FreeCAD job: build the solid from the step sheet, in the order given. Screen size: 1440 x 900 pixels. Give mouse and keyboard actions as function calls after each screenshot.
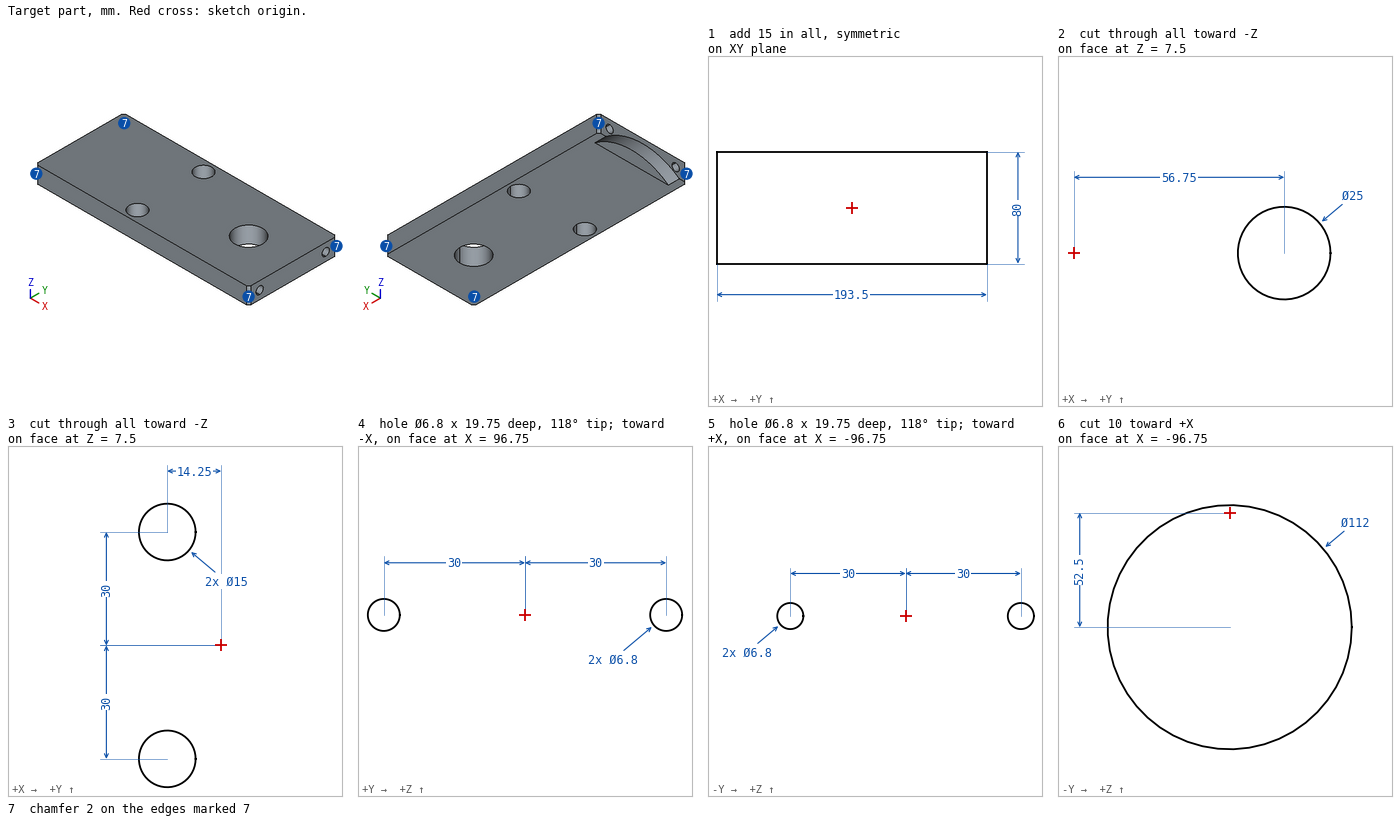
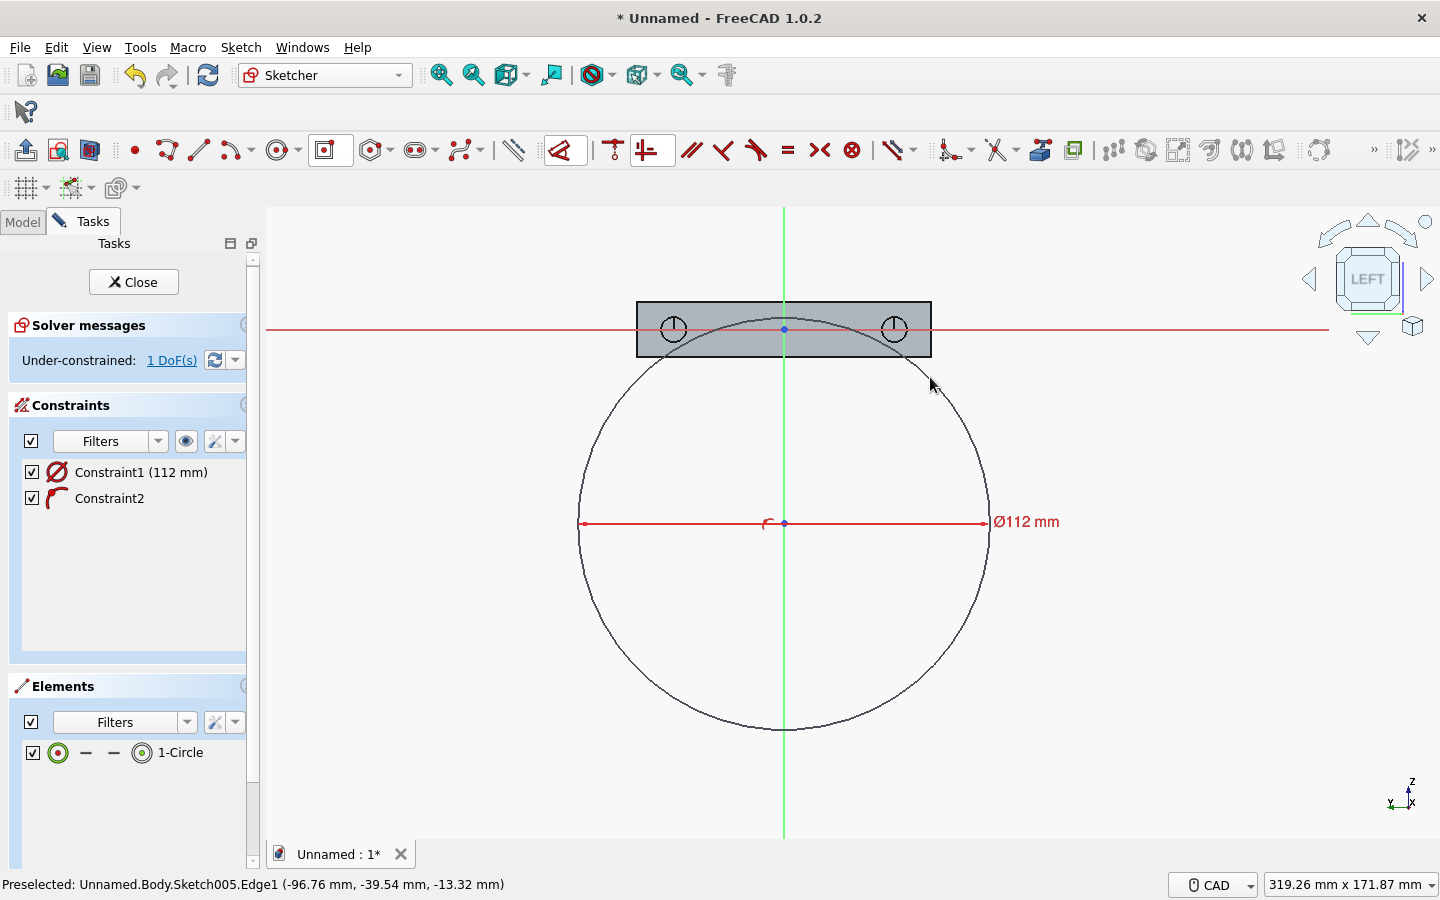
click(784, 524)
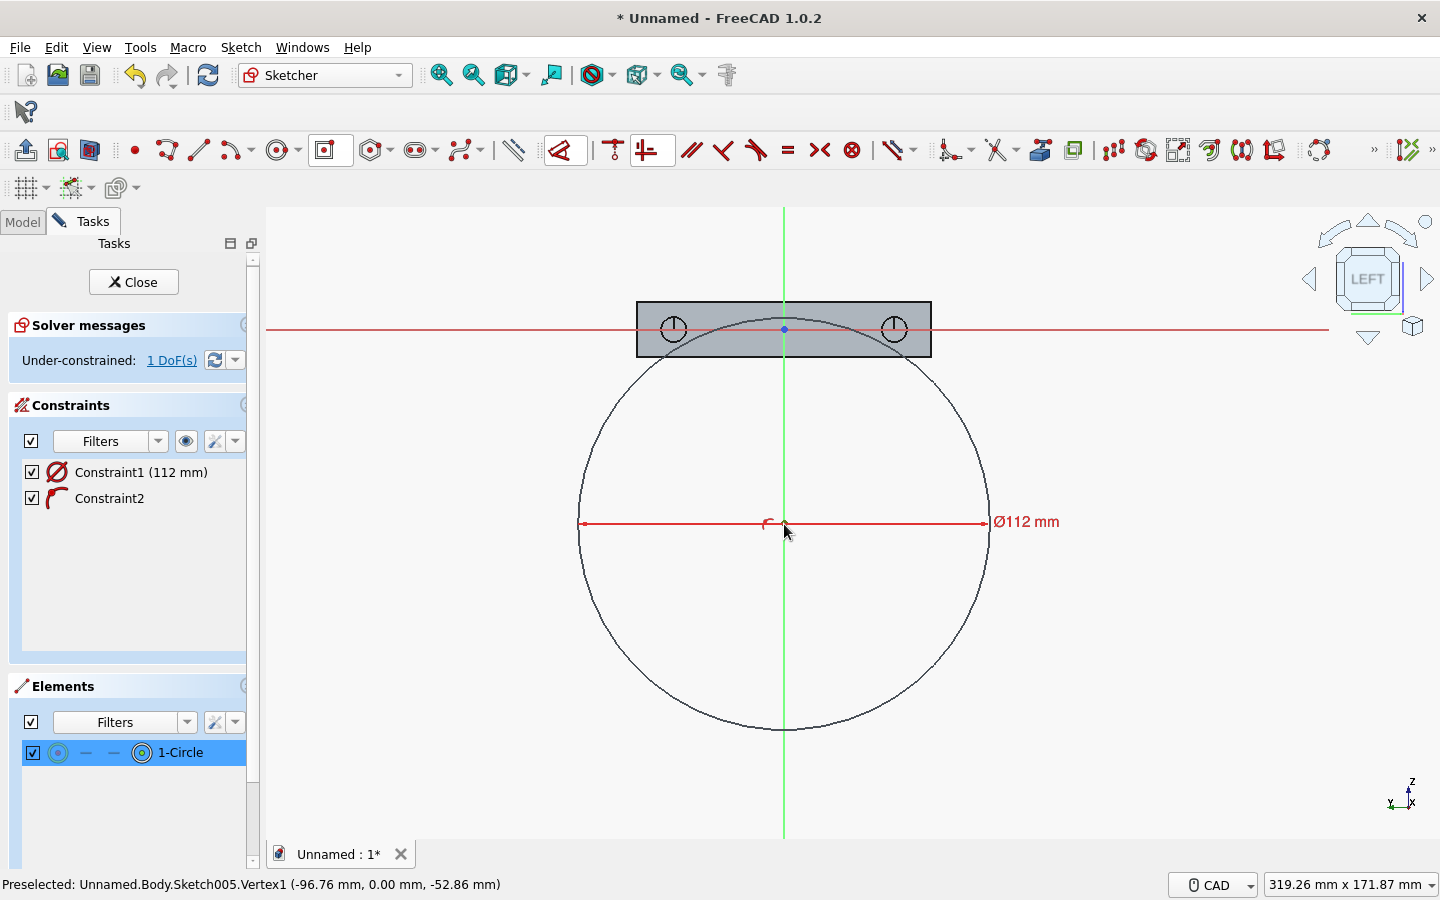
click(582, 150)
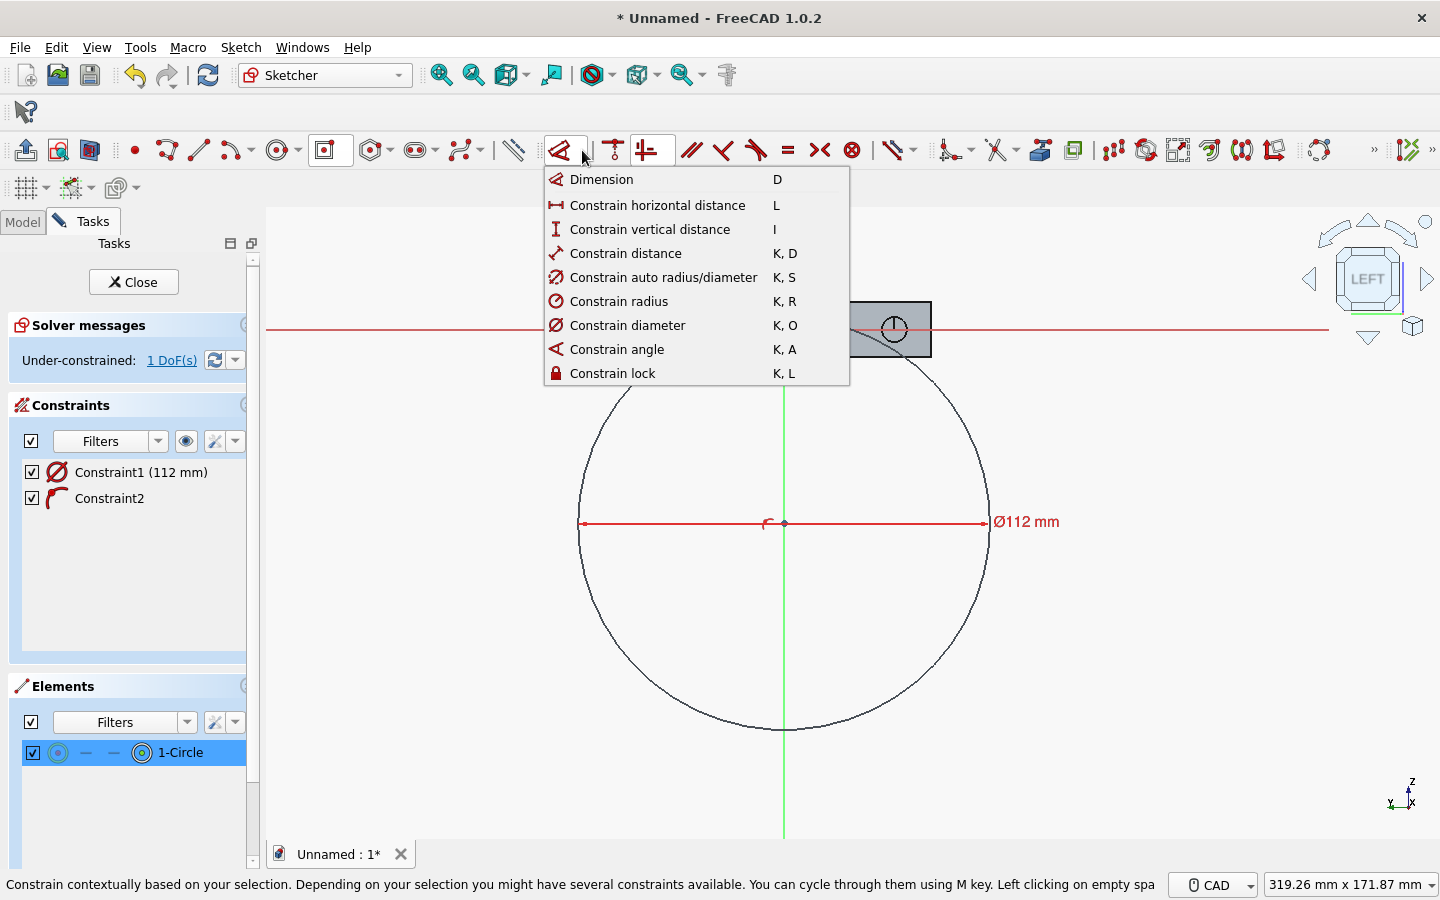
click(697, 229)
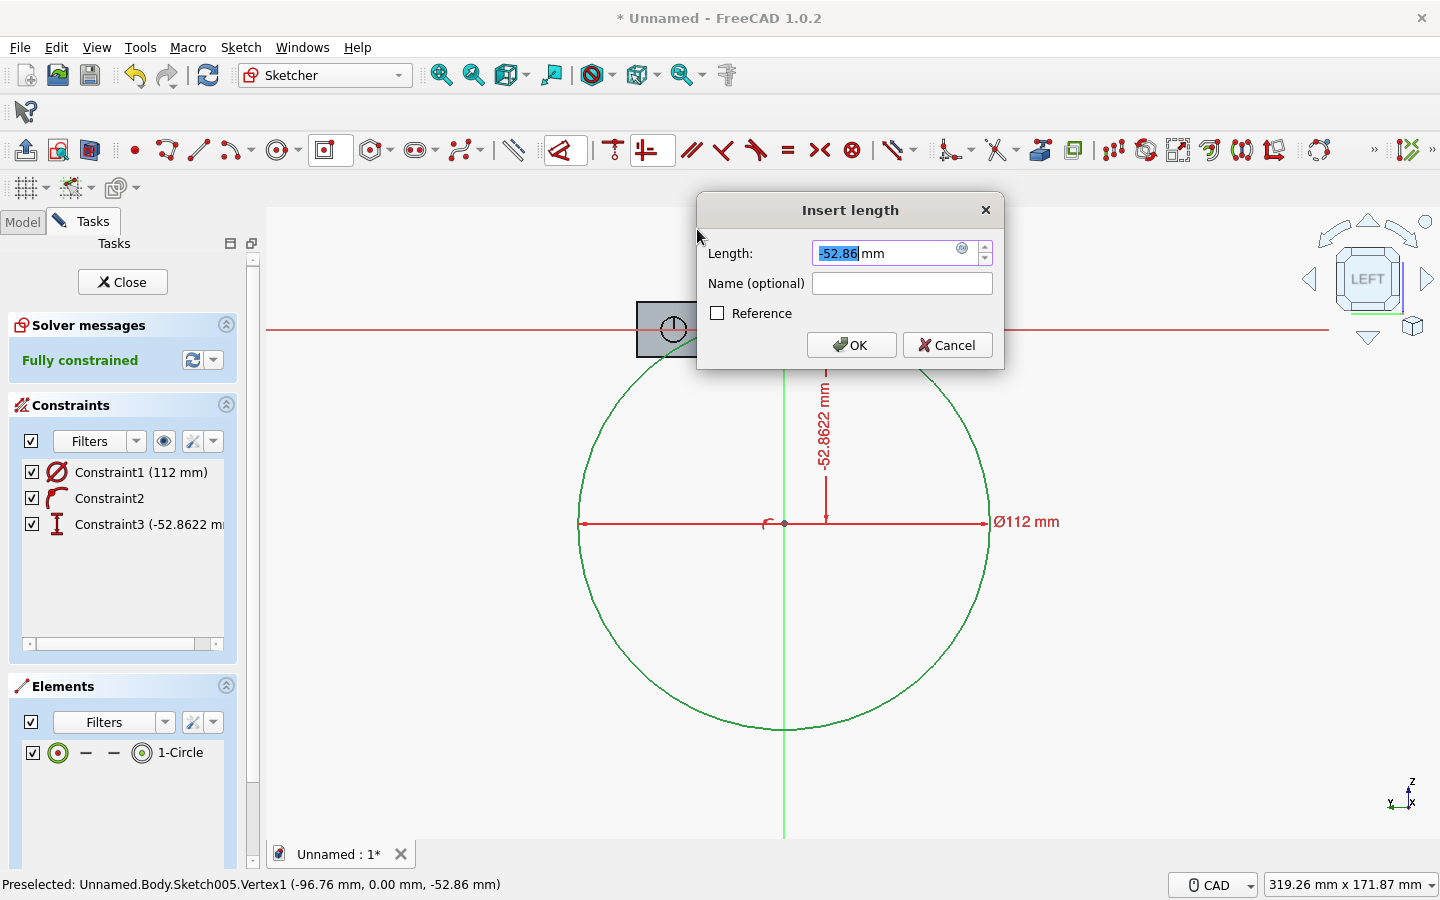
text(-52.5)
key(Return)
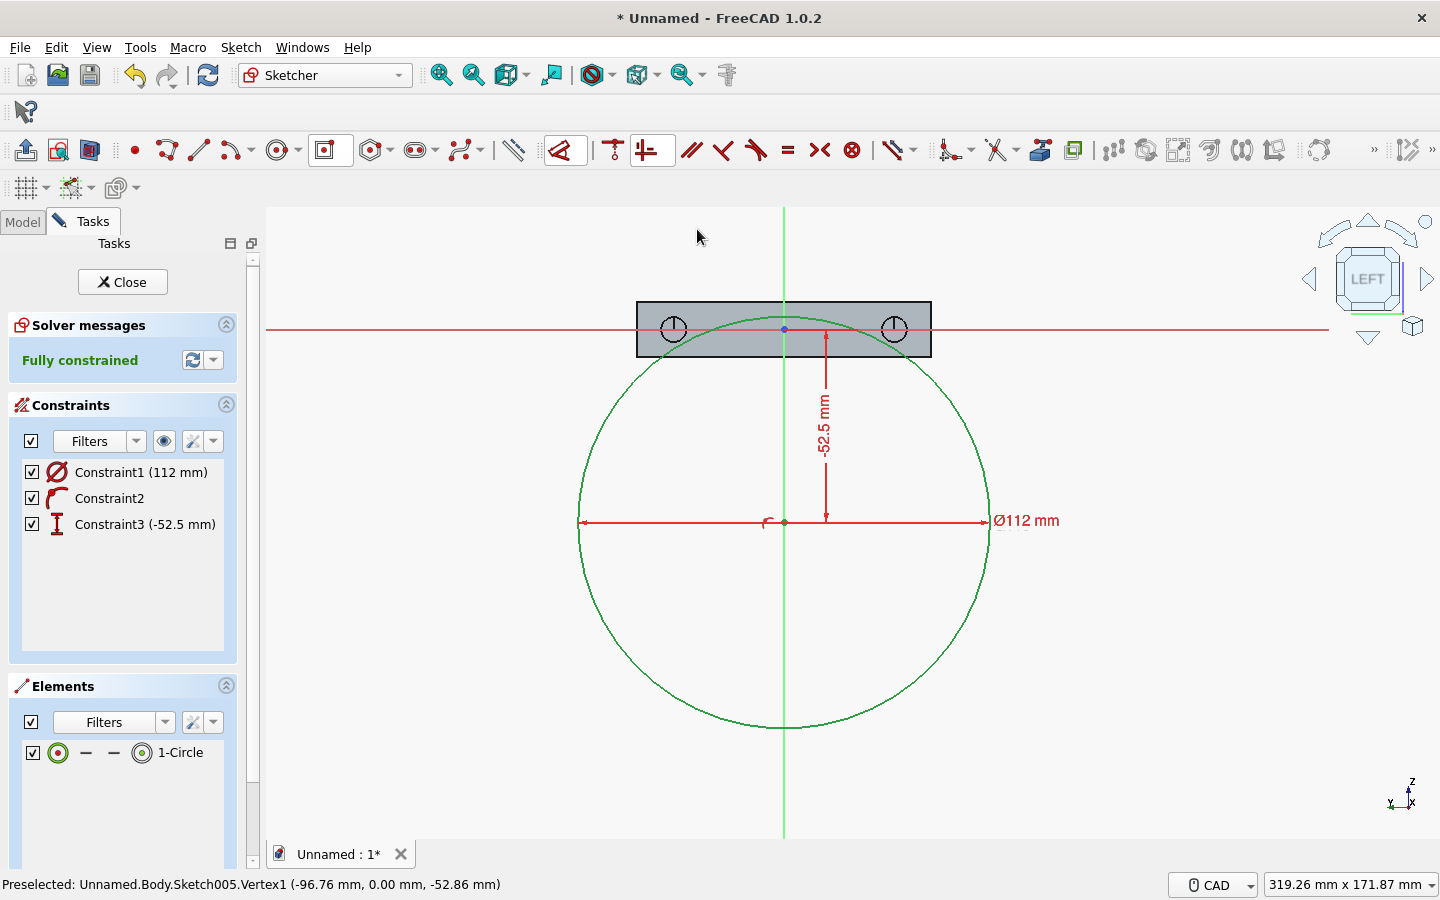
click(123, 282)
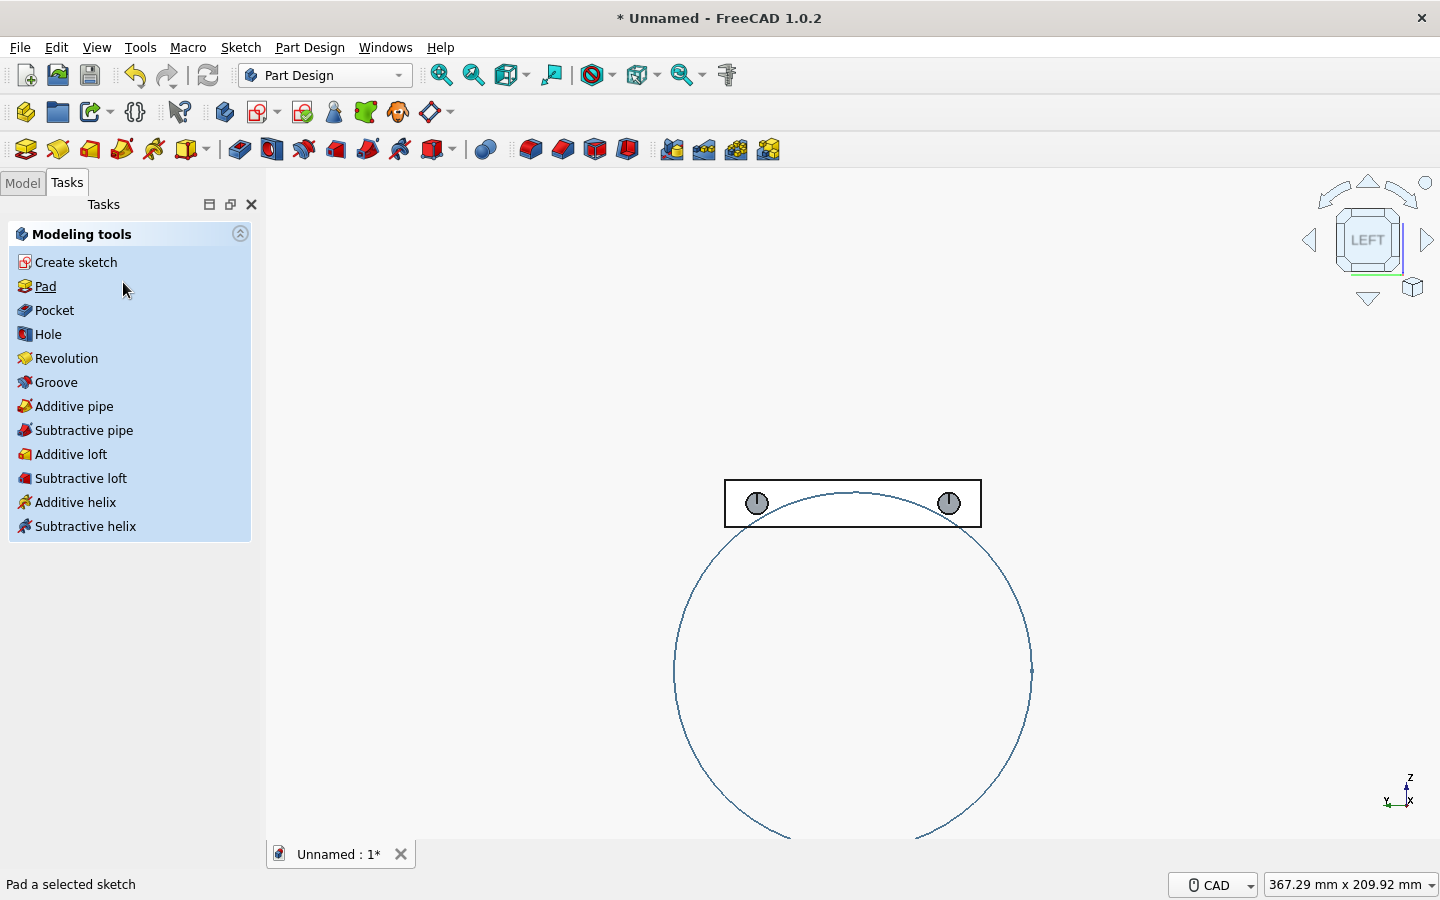
click(240, 150)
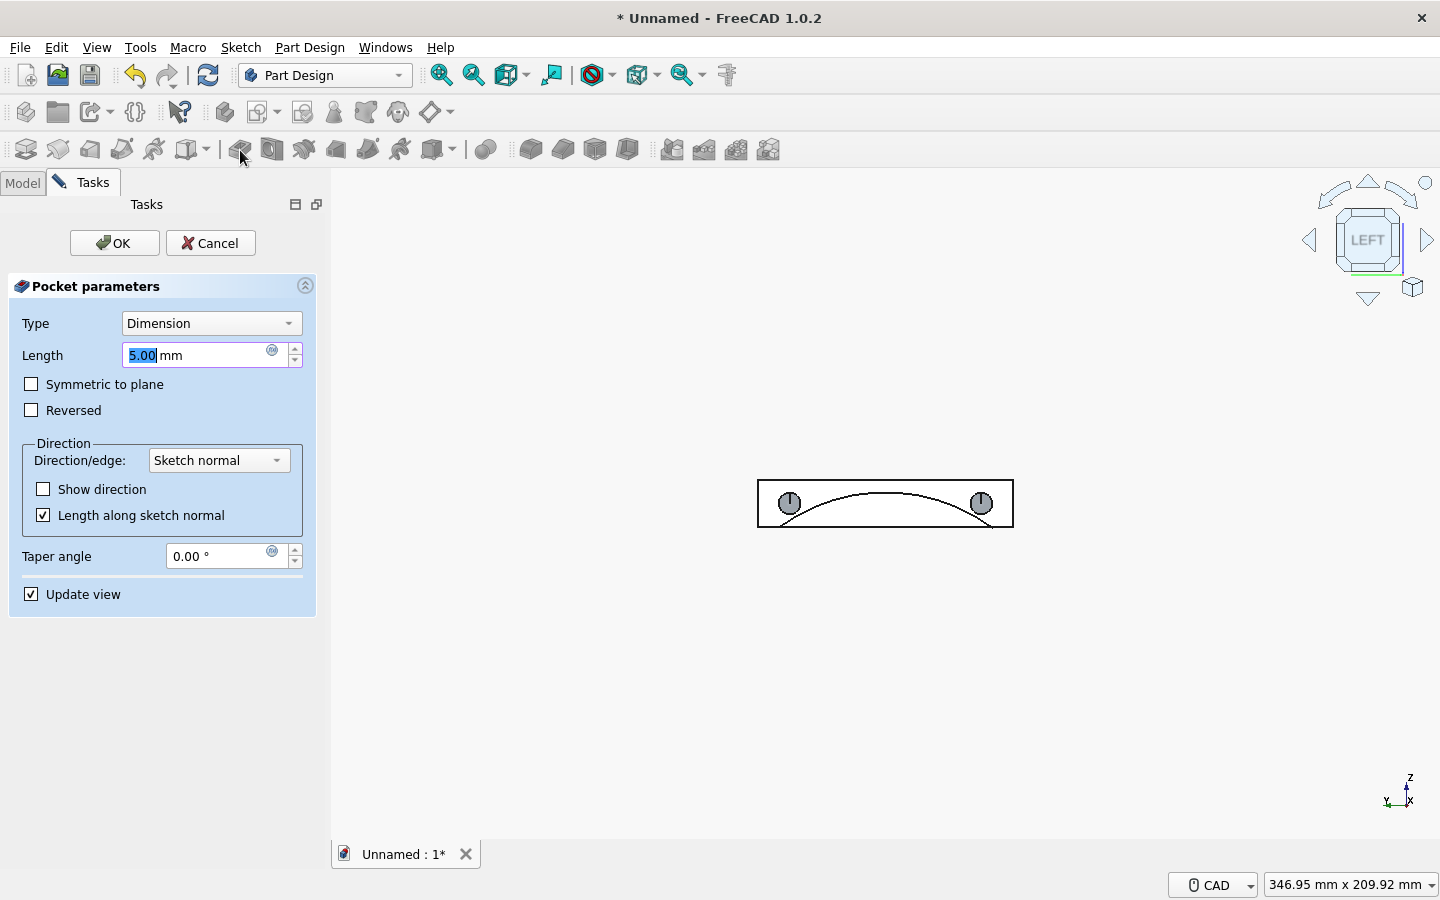
text(10)
key(Tab)